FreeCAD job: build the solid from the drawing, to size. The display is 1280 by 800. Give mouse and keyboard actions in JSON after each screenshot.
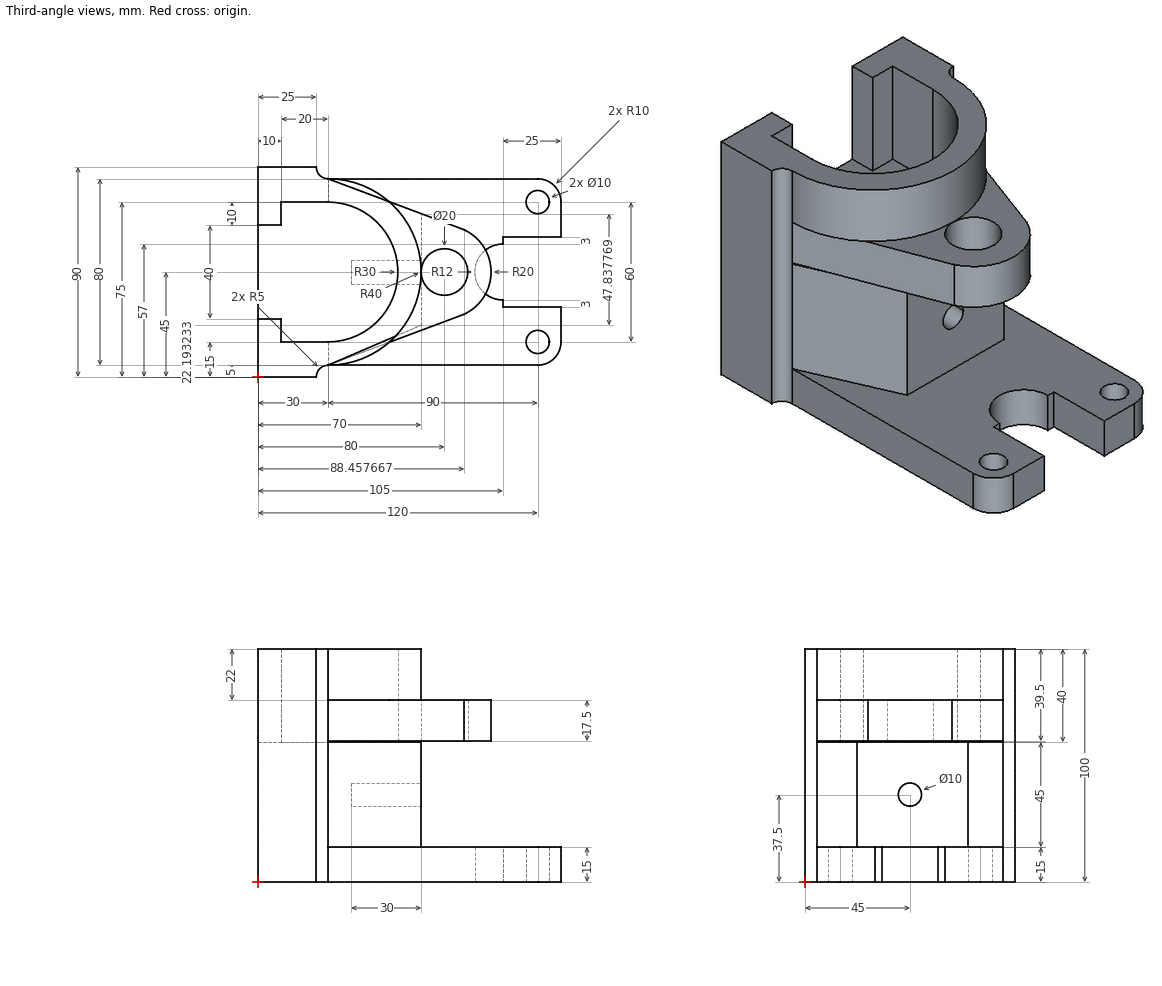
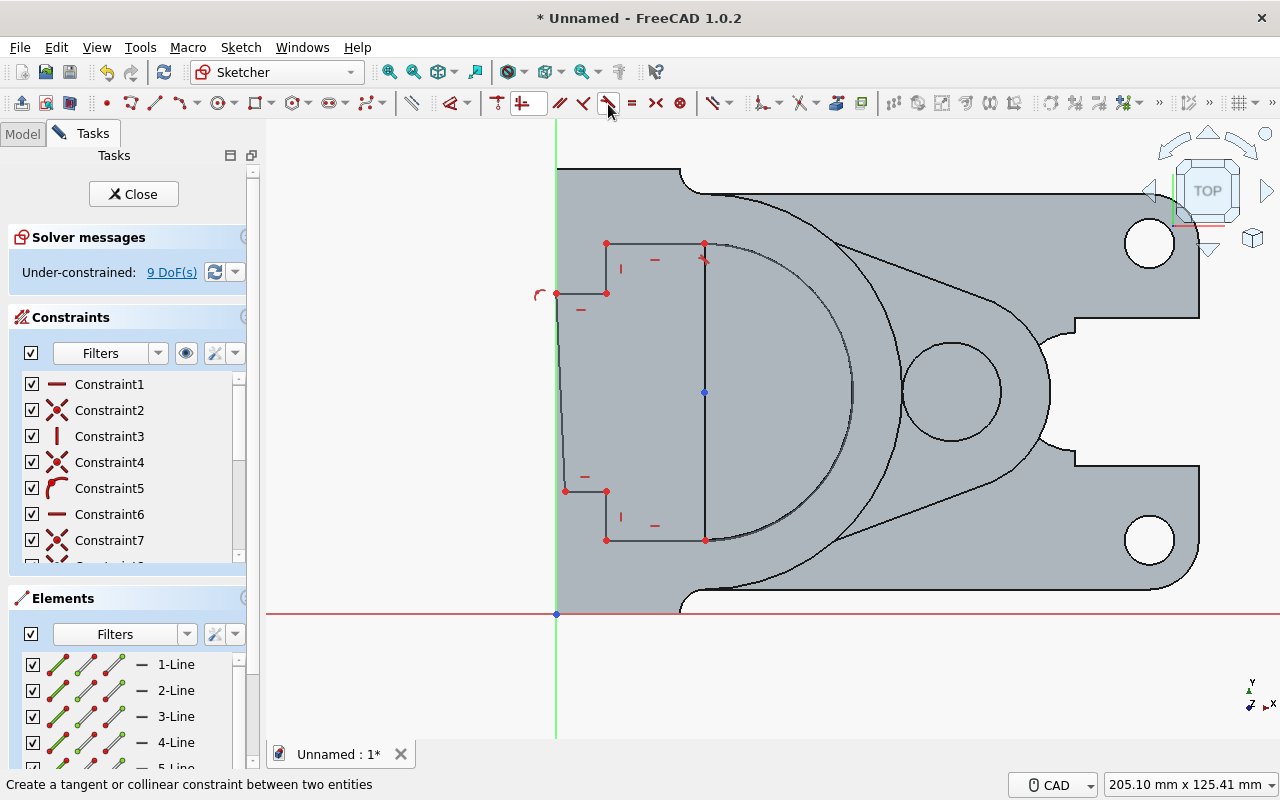
{"action": "left_click", "coordinate": [636, 541]}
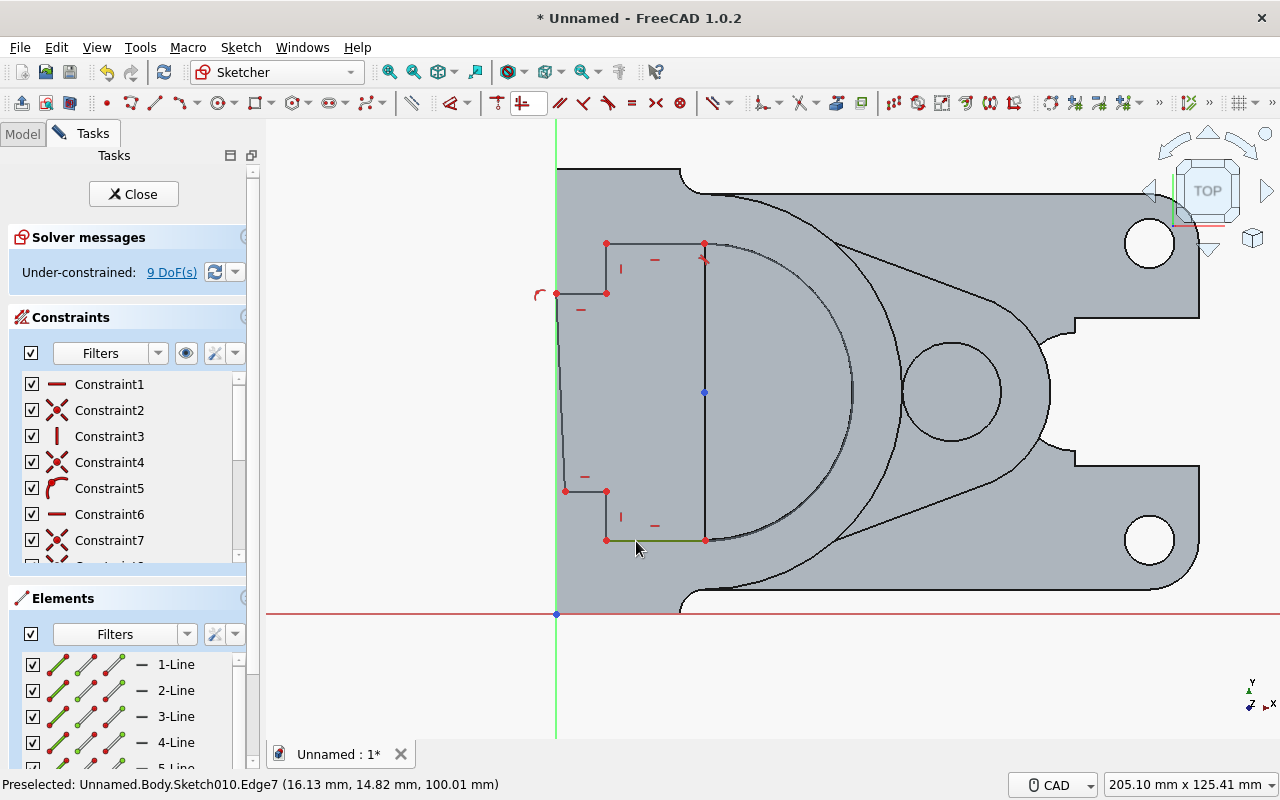
{"action": "left_click", "coordinate": [825, 480]}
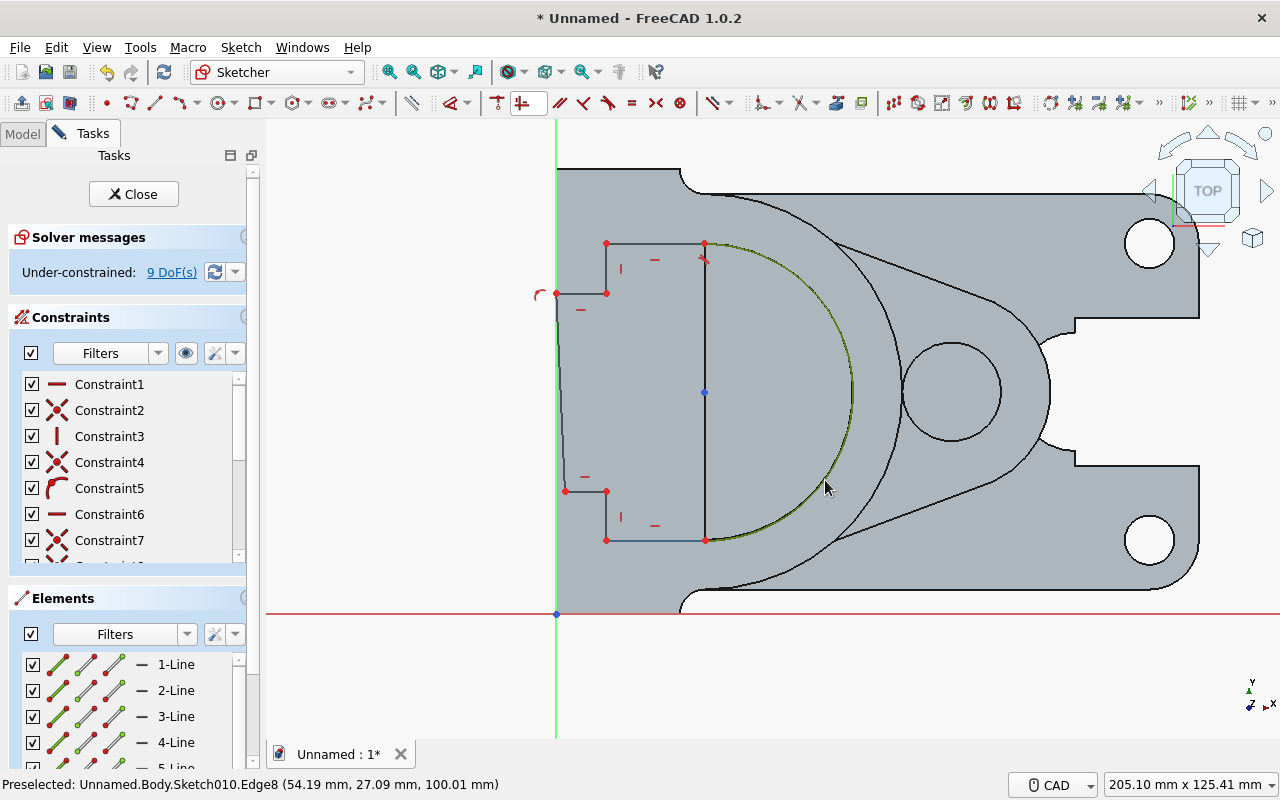
{"action": "left_click", "coordinate": [608, 104]}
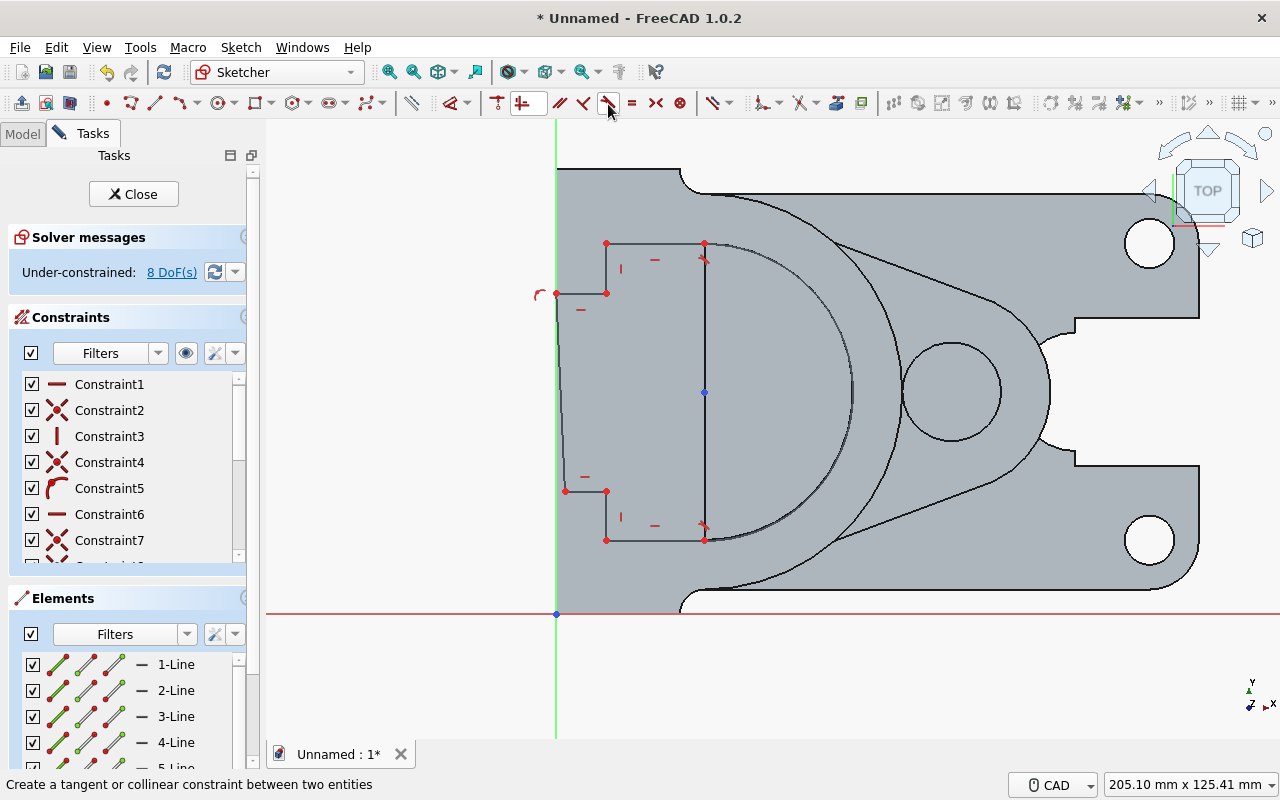
{"action": "left_click", "coordinate": [559, 353]}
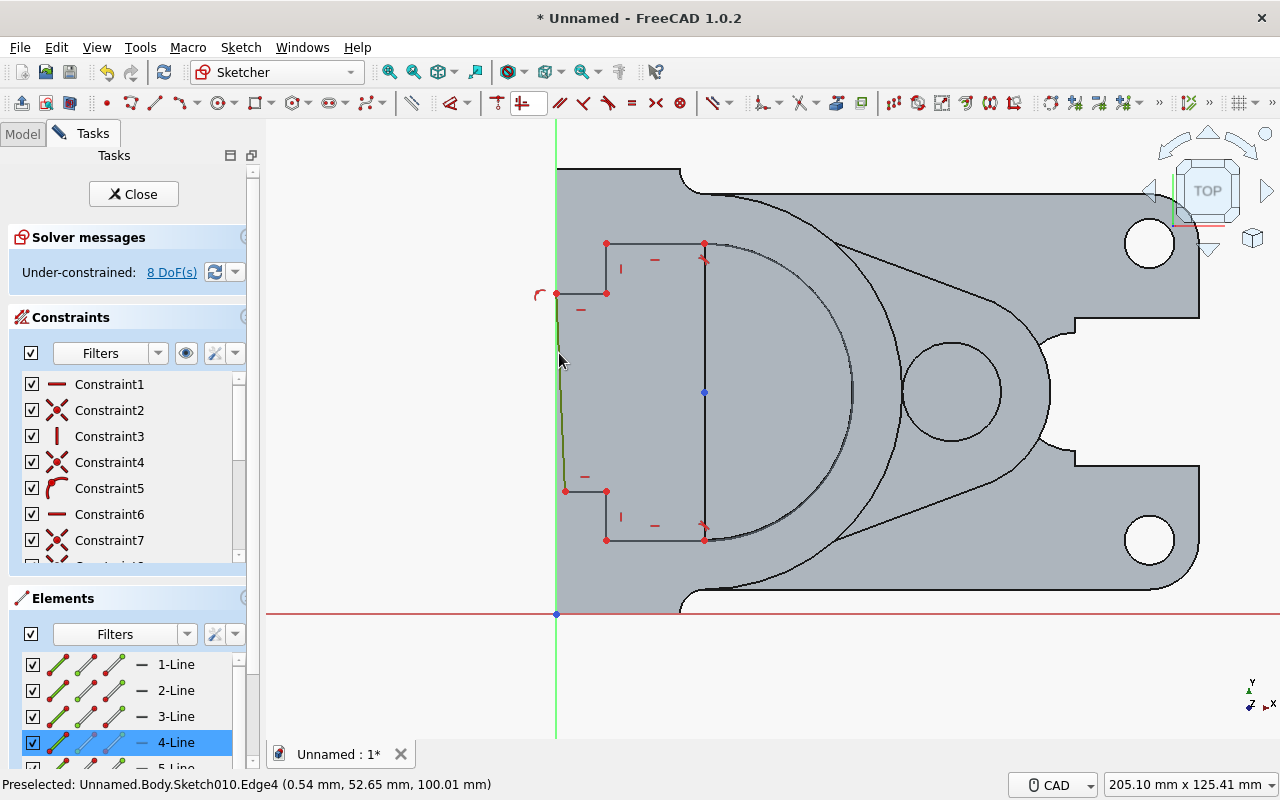
{"action": "key", "text": "v"}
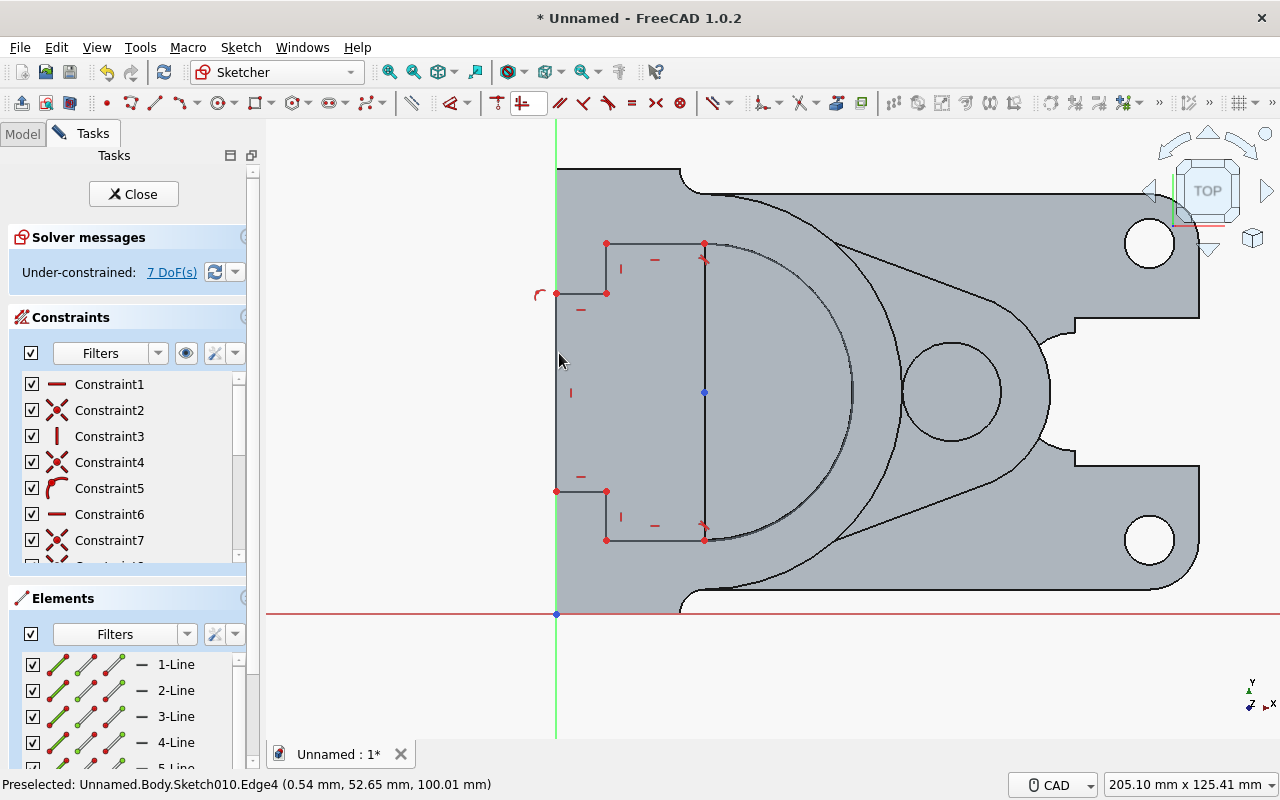
{"action": "key", "text": "d"}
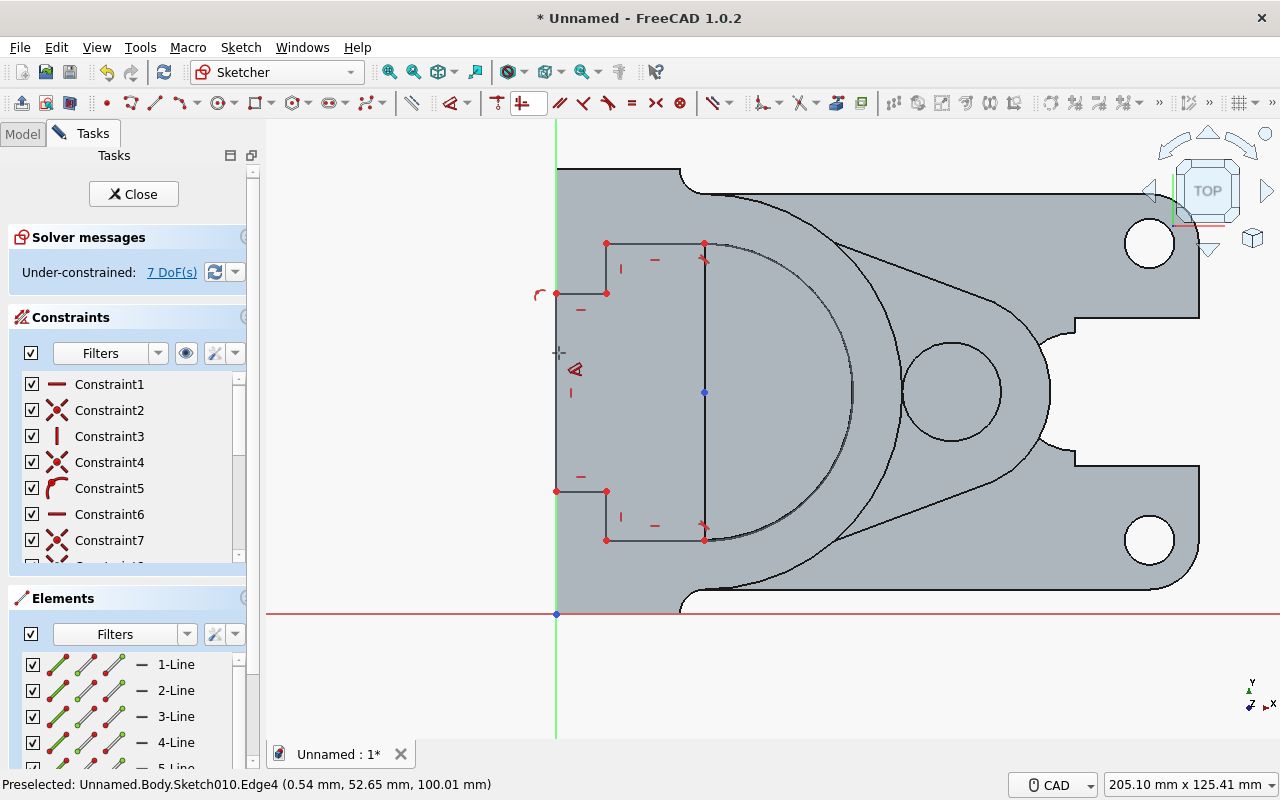
{"action": "left_click", "coordinate": [825, 480]}
{"action": "left_click", "coordinate": [851, 499]}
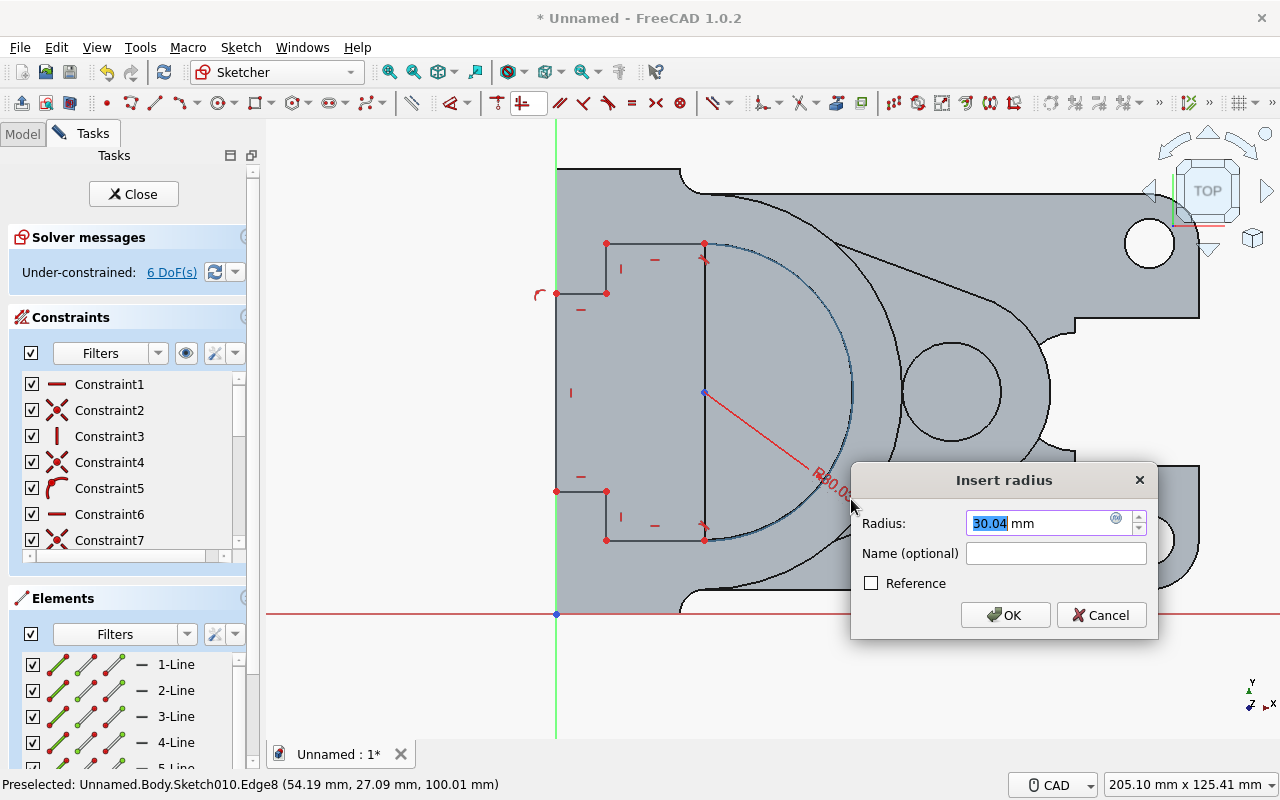
{"action": "type", "text": "30"}
{"action": "key", "text": "Return"}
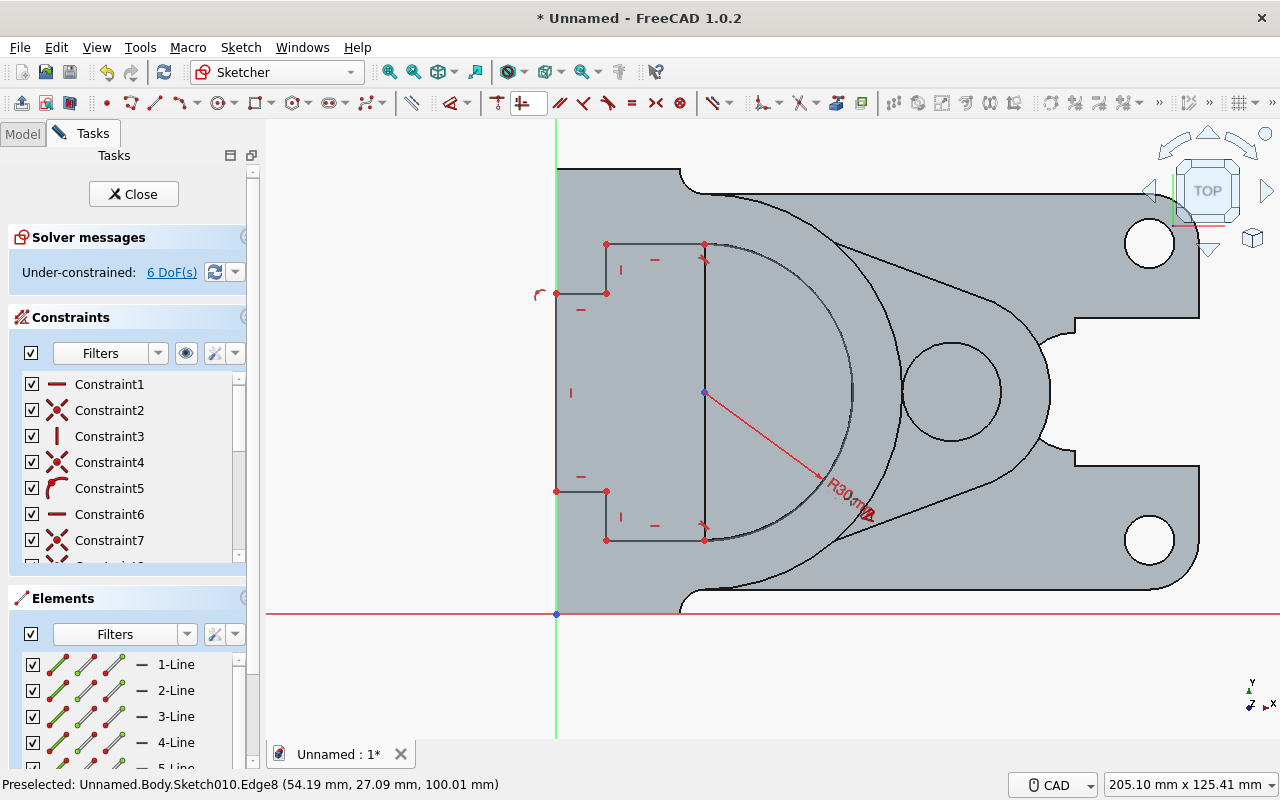
{"action": "left_click", "coordinate": [675, 244]}
{"action": "left_click", "coordinate": [655, 210]}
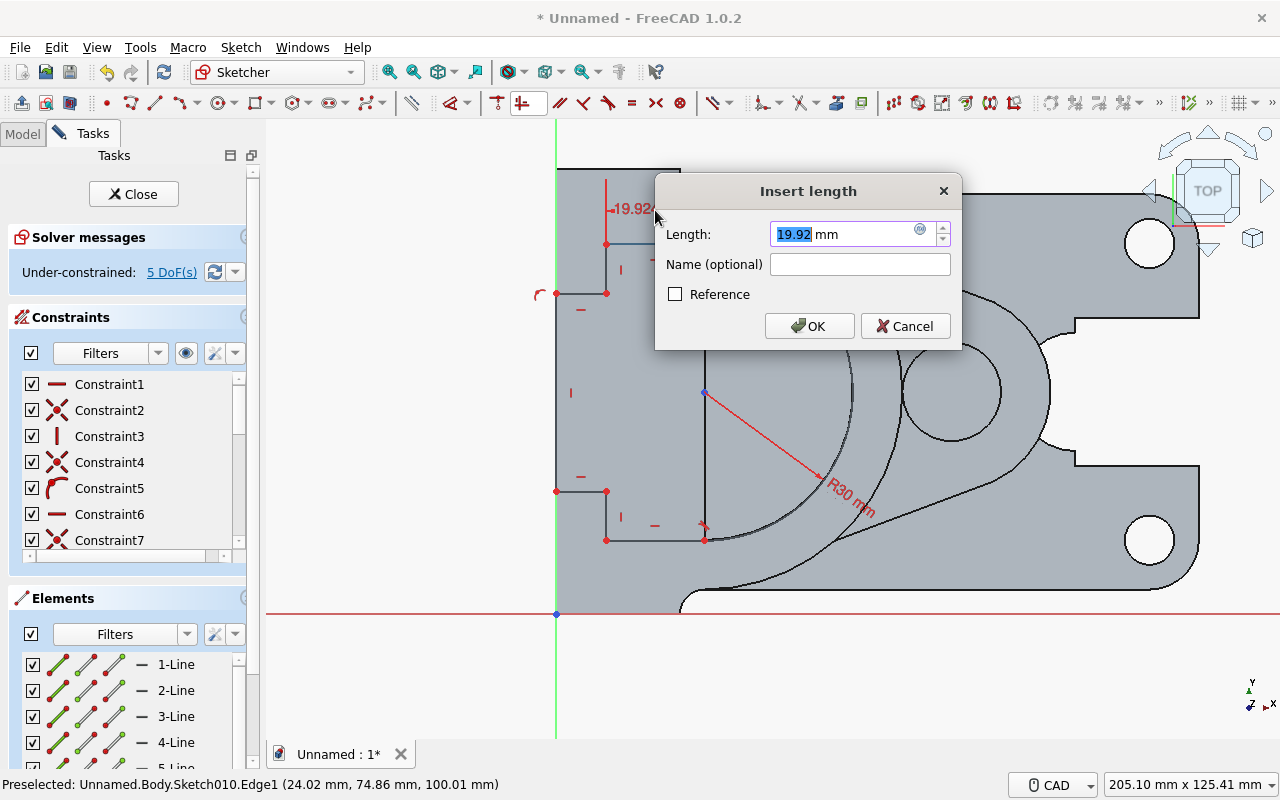
{"action": "type", "text": "20"}
{"action": "key", "text": "Return"}